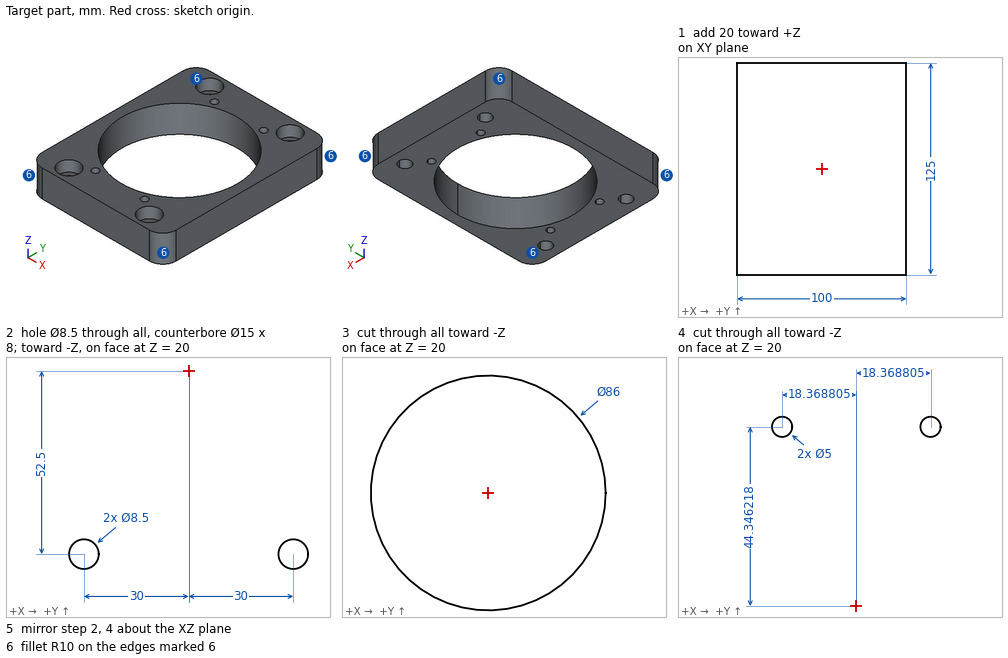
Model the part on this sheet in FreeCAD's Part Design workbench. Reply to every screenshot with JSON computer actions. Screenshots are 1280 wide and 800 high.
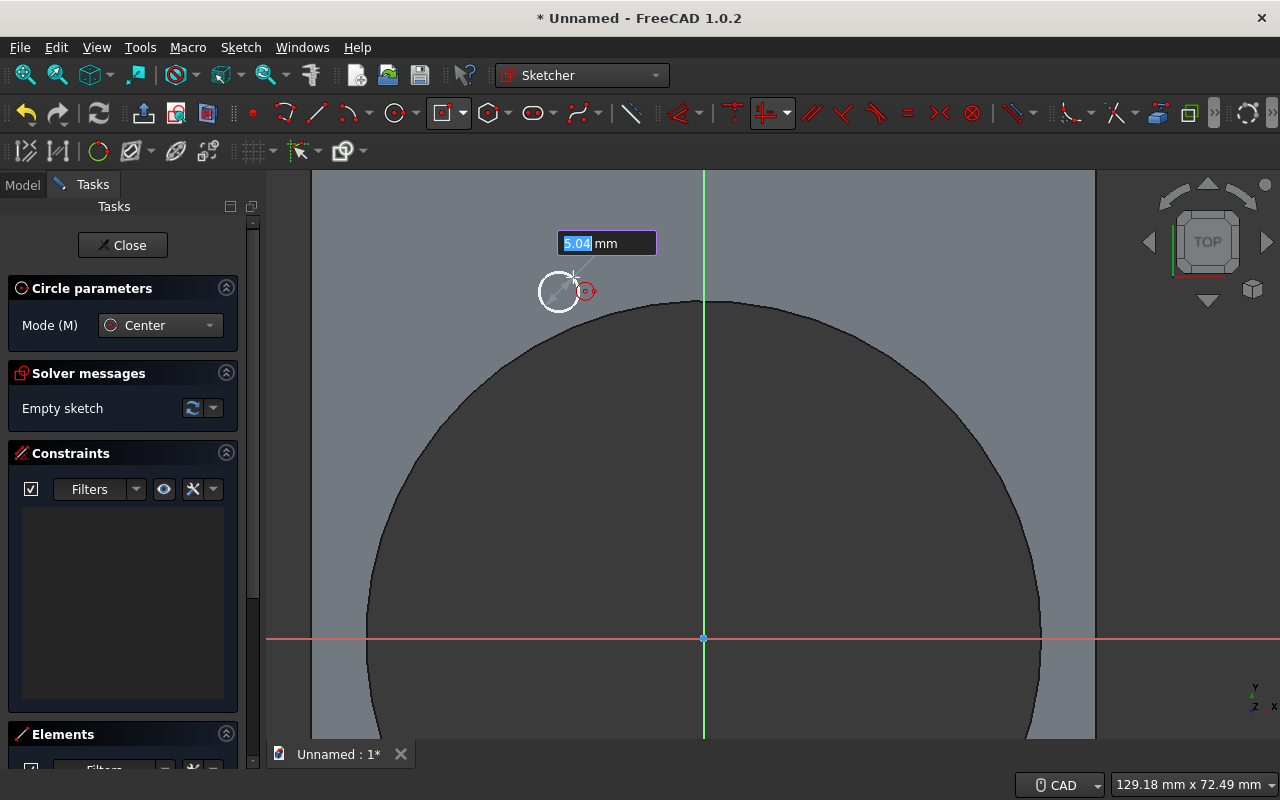
{"action": "type", "text": "5"}
{"action": "key", "text": "Return"}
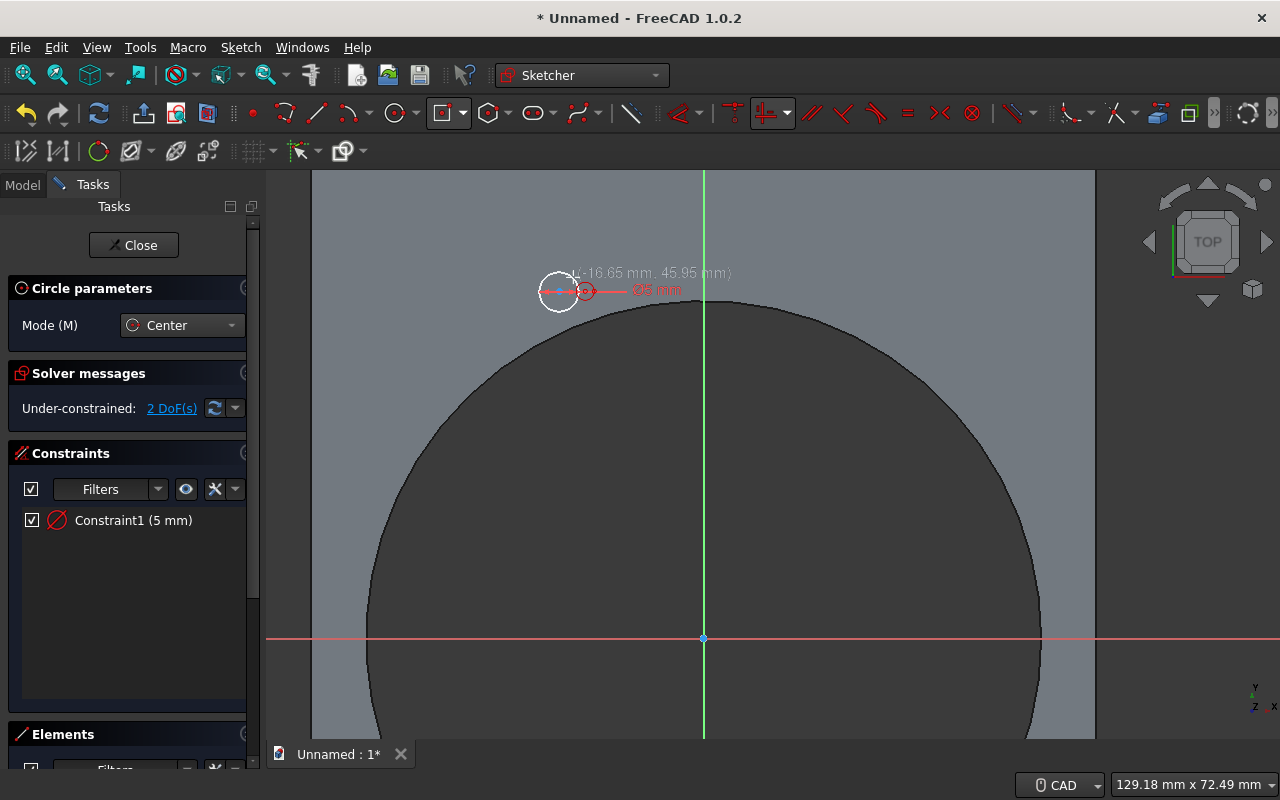
{"action": "left_click", "coordinate": [848, 291]}
{"action": "mouse_move", "coordinate": [862, 277]}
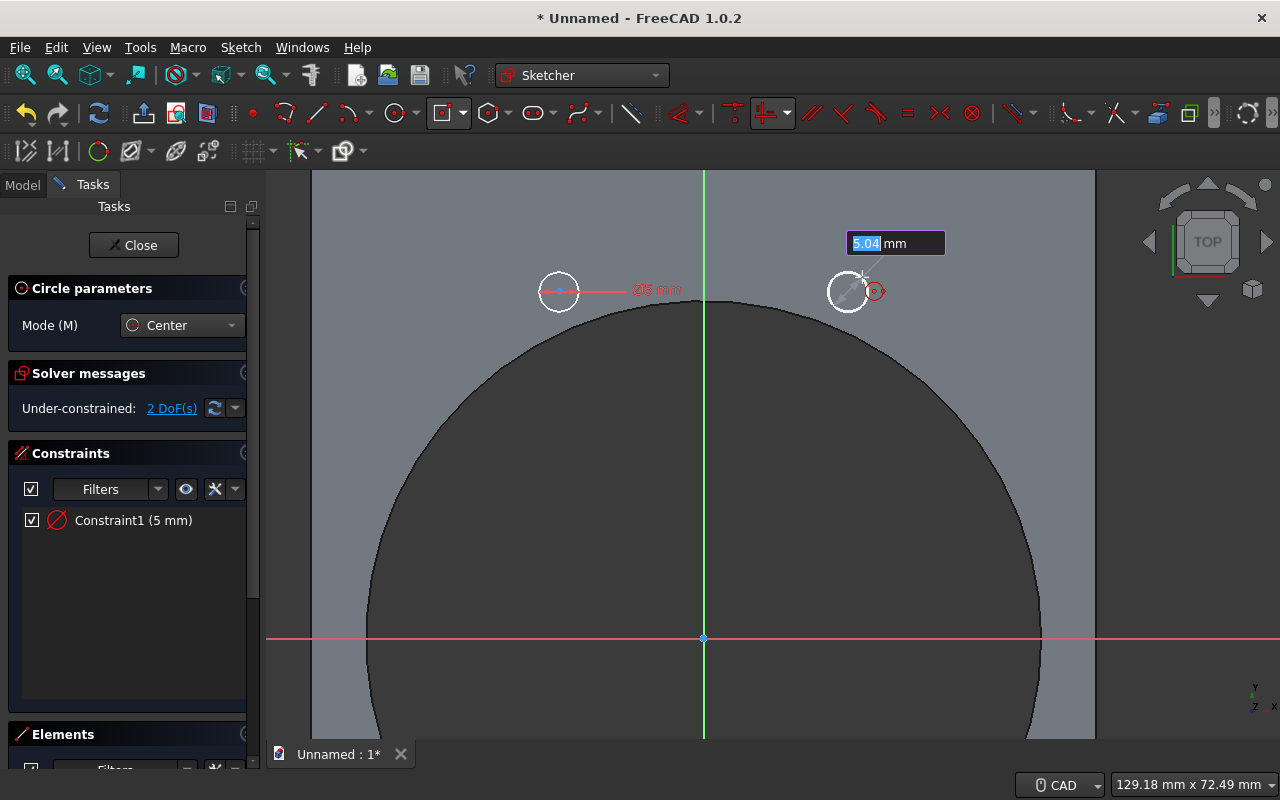
{"action": "type", "text": "5"}
{"action": "key", "text": "Return"}
{"action": "key", "text": "Escape"}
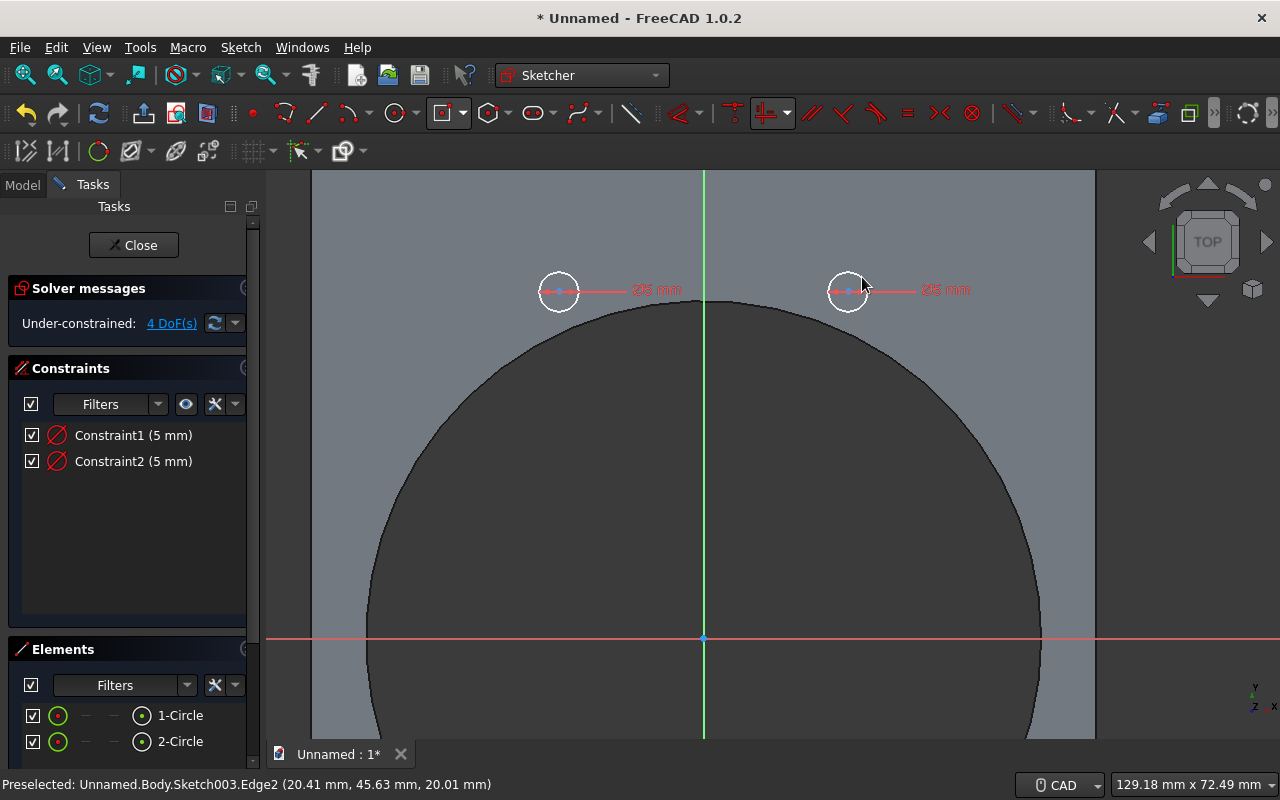
{"action": "left_click", "coordinate": [559, 292]}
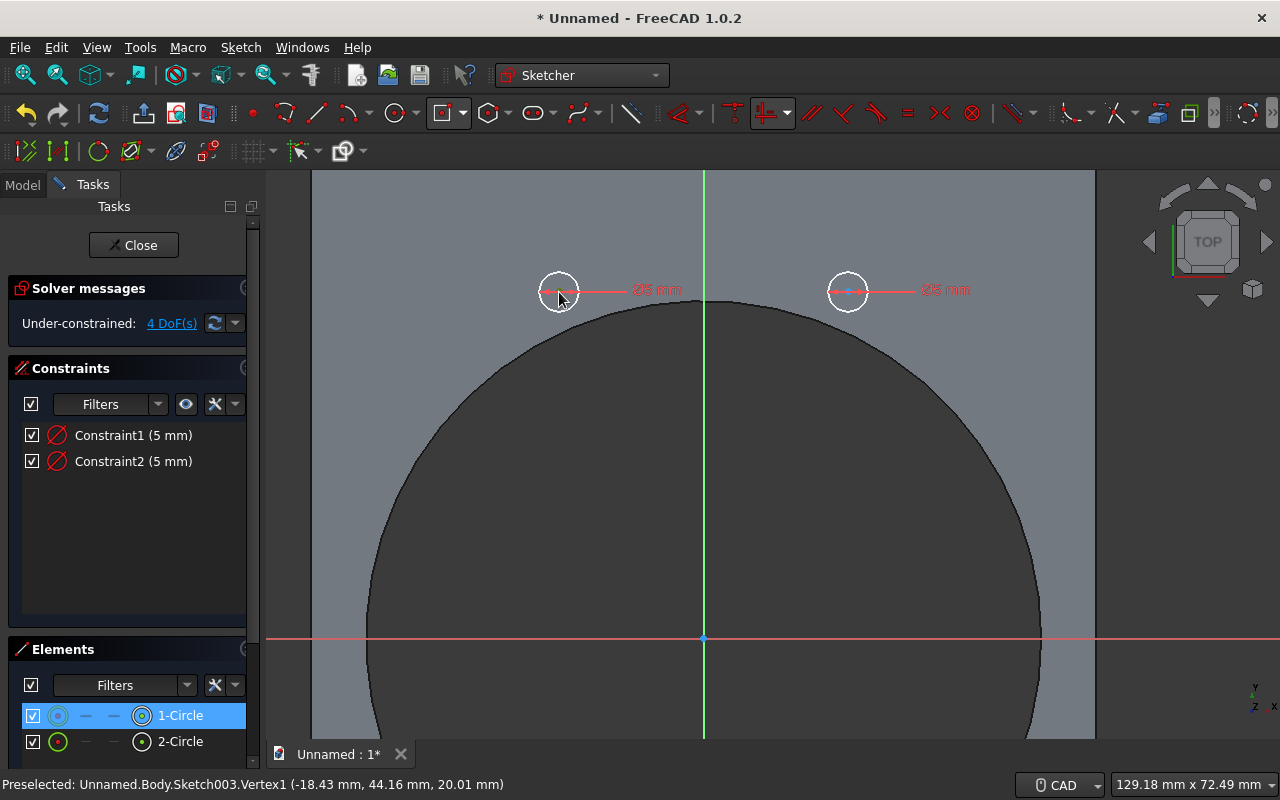
{"action": "left_click", "coordinate": [848, 292]}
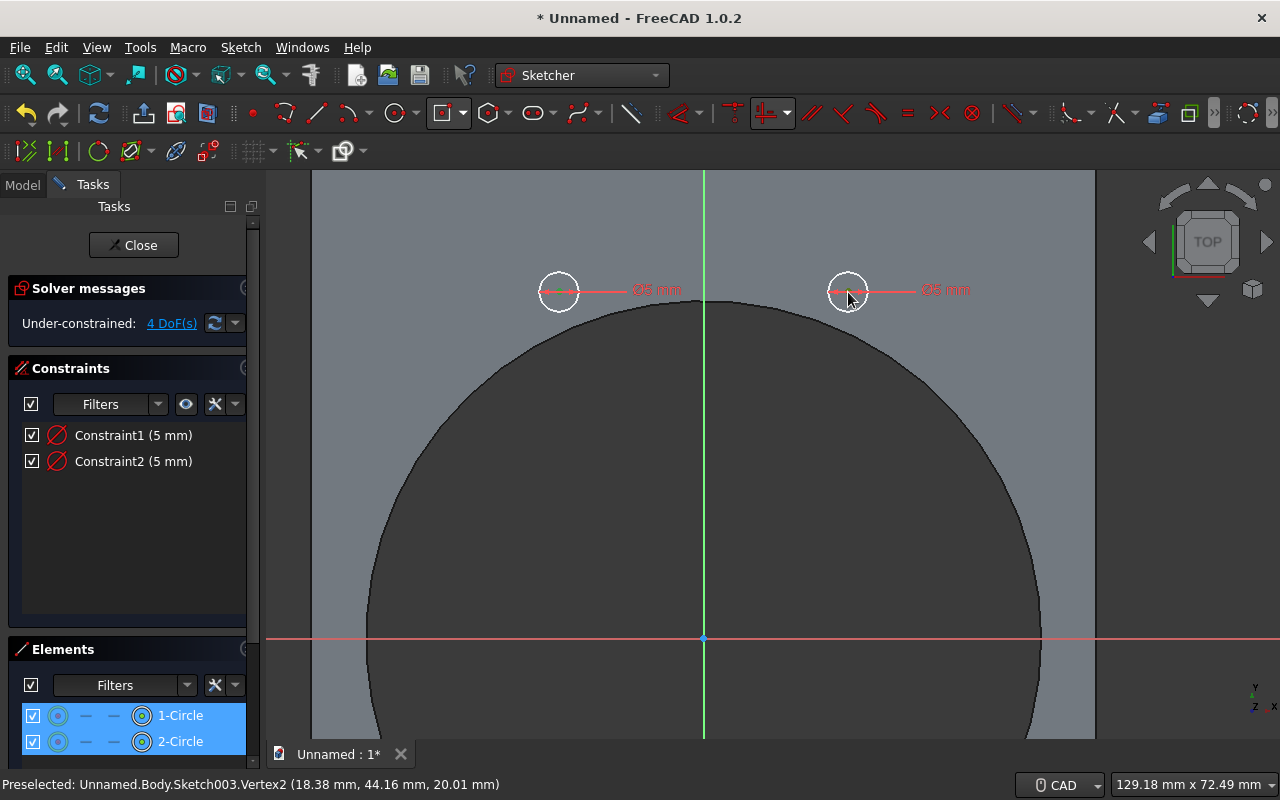
{"action": "left_click", "coordinate": [790, 114]}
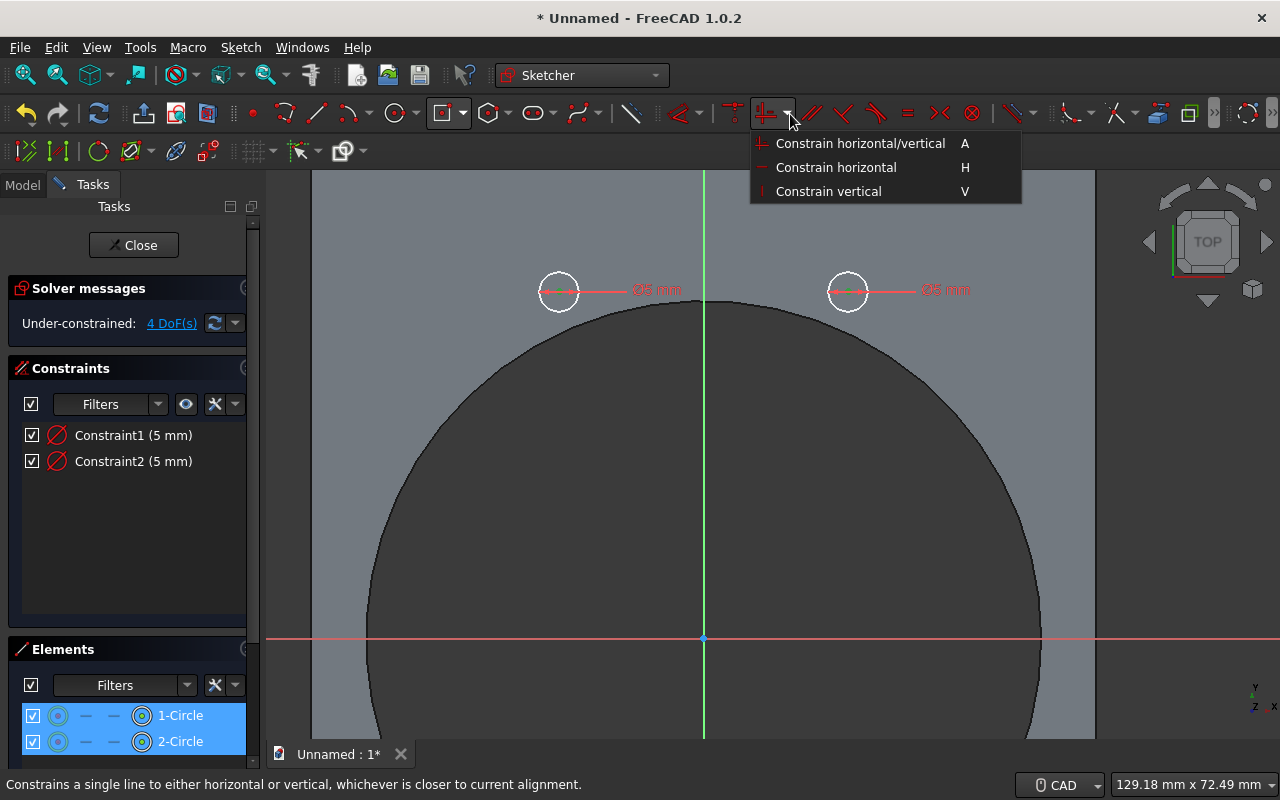
{"action": "left_click", "coordinate": [886, 167]}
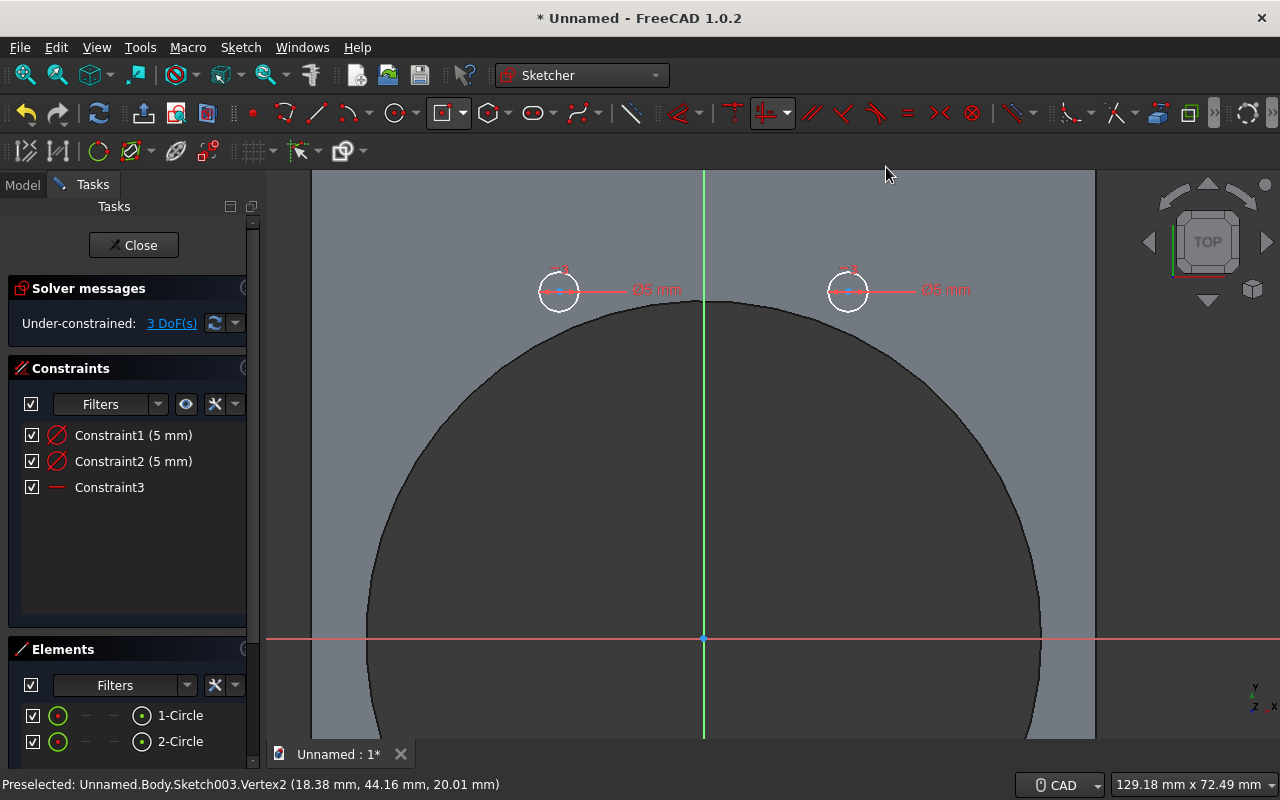
{"action": "left_click", "coordinate": [678, 114]}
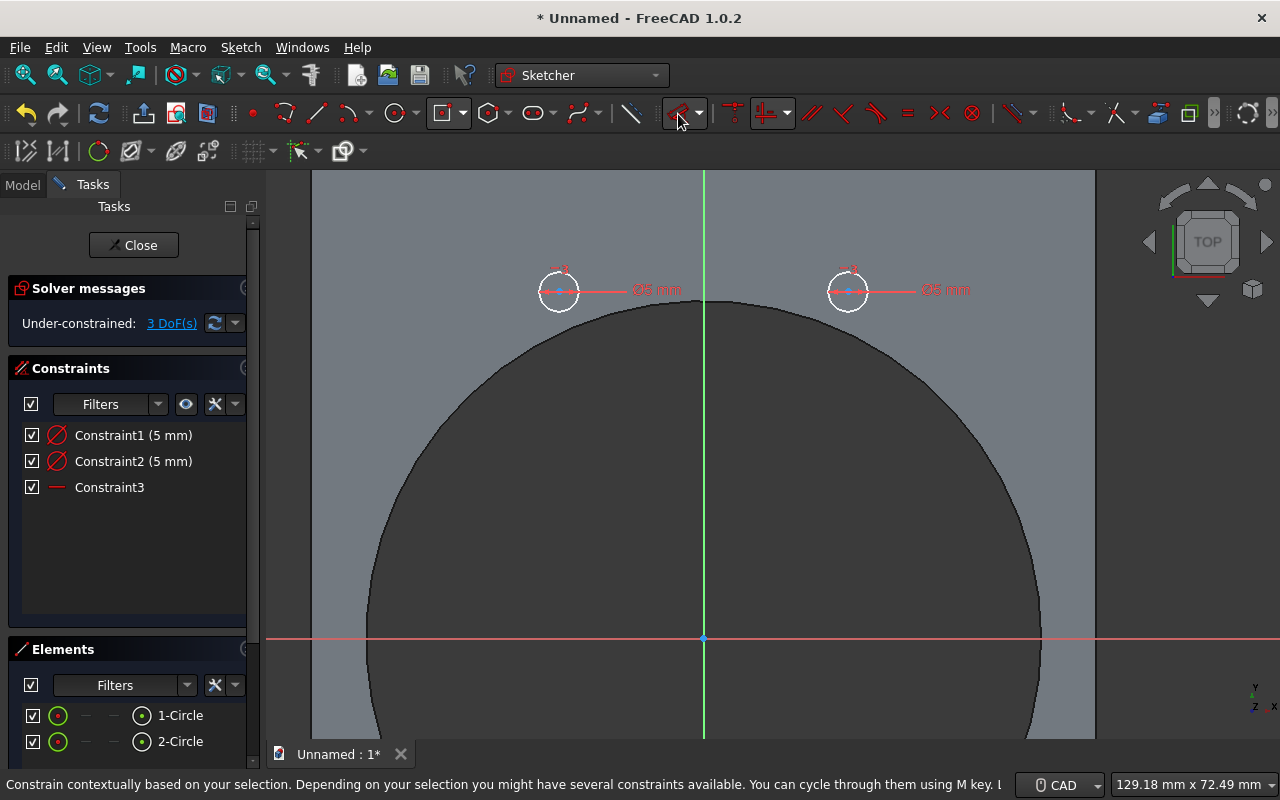
{"action": "left_click", "coordinate": [559, 292]}
{"action": "left_click", "coordinate": [631, 673]}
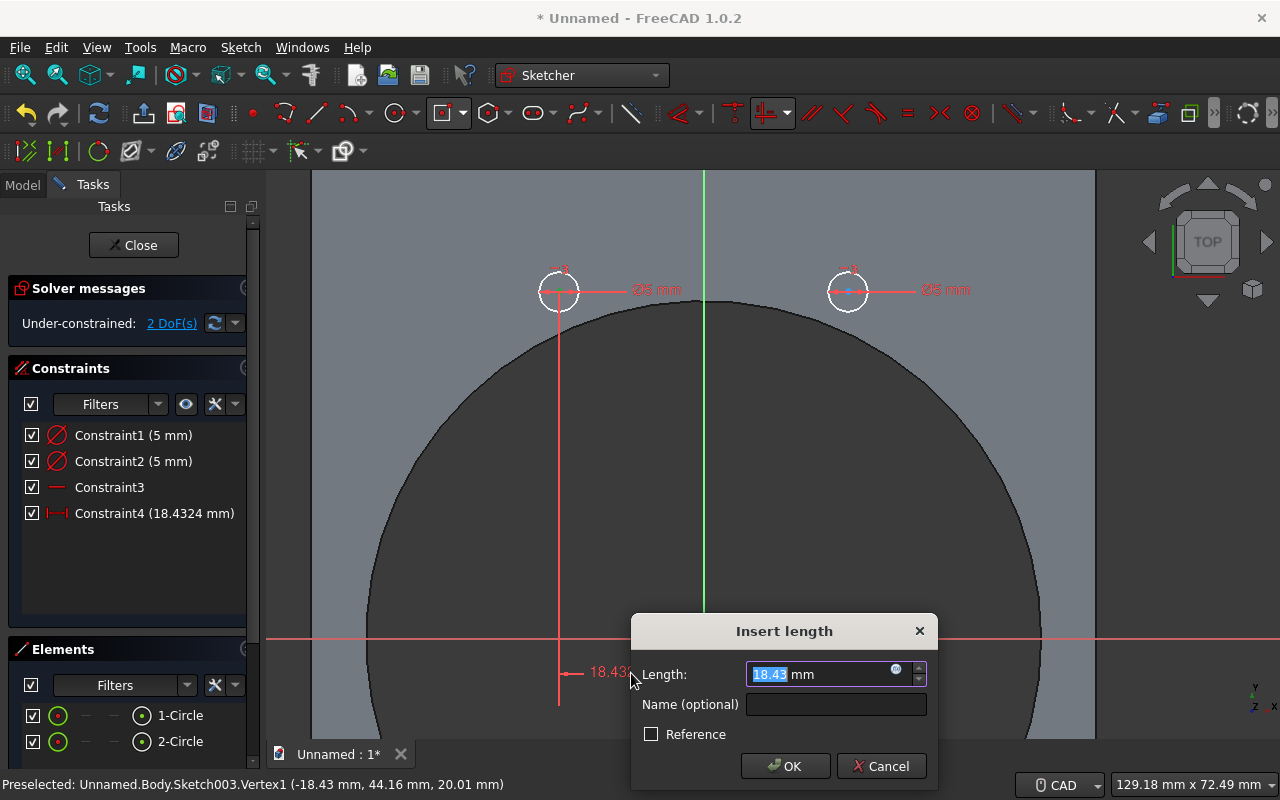
{"action": "type", "text": "18.368805"}
{"action": "key", "text": "Return"}